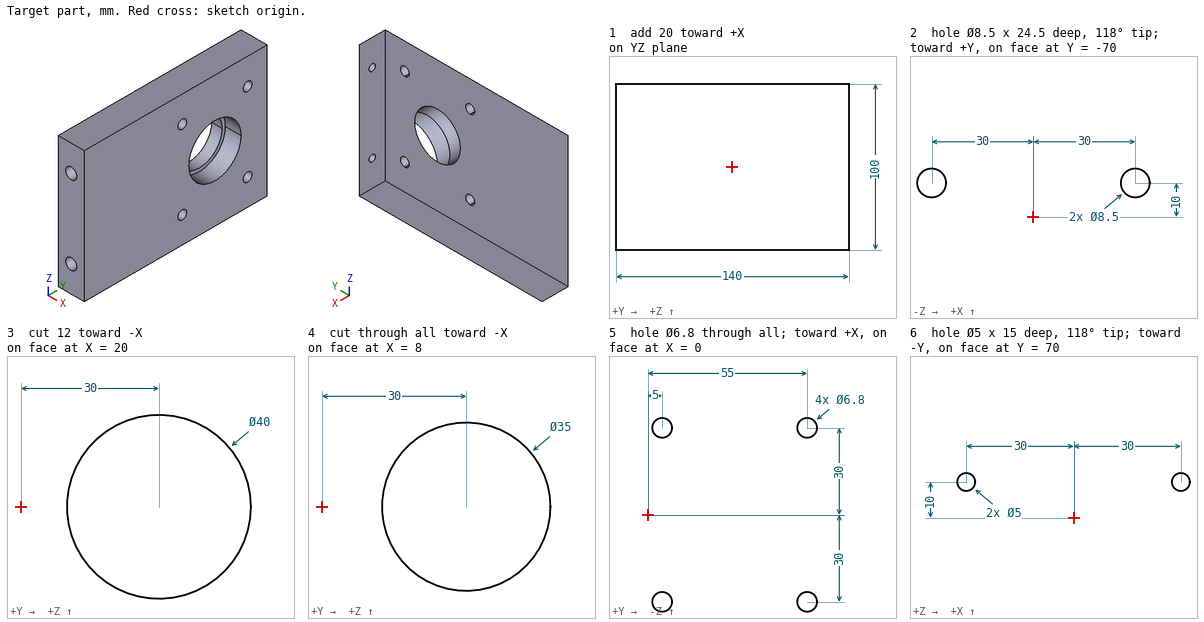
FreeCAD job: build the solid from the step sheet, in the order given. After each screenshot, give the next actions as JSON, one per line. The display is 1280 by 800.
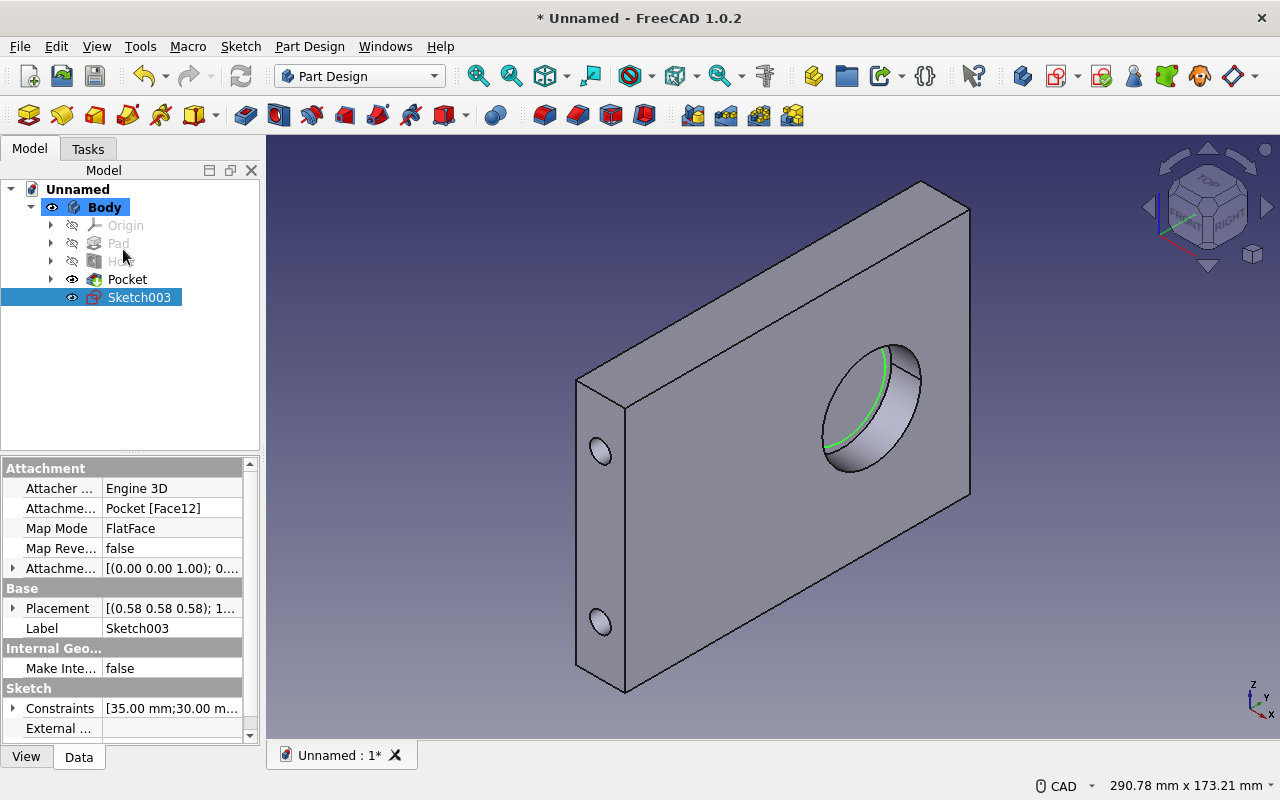
{"action": "left_click", "coordinate": [246, 116]}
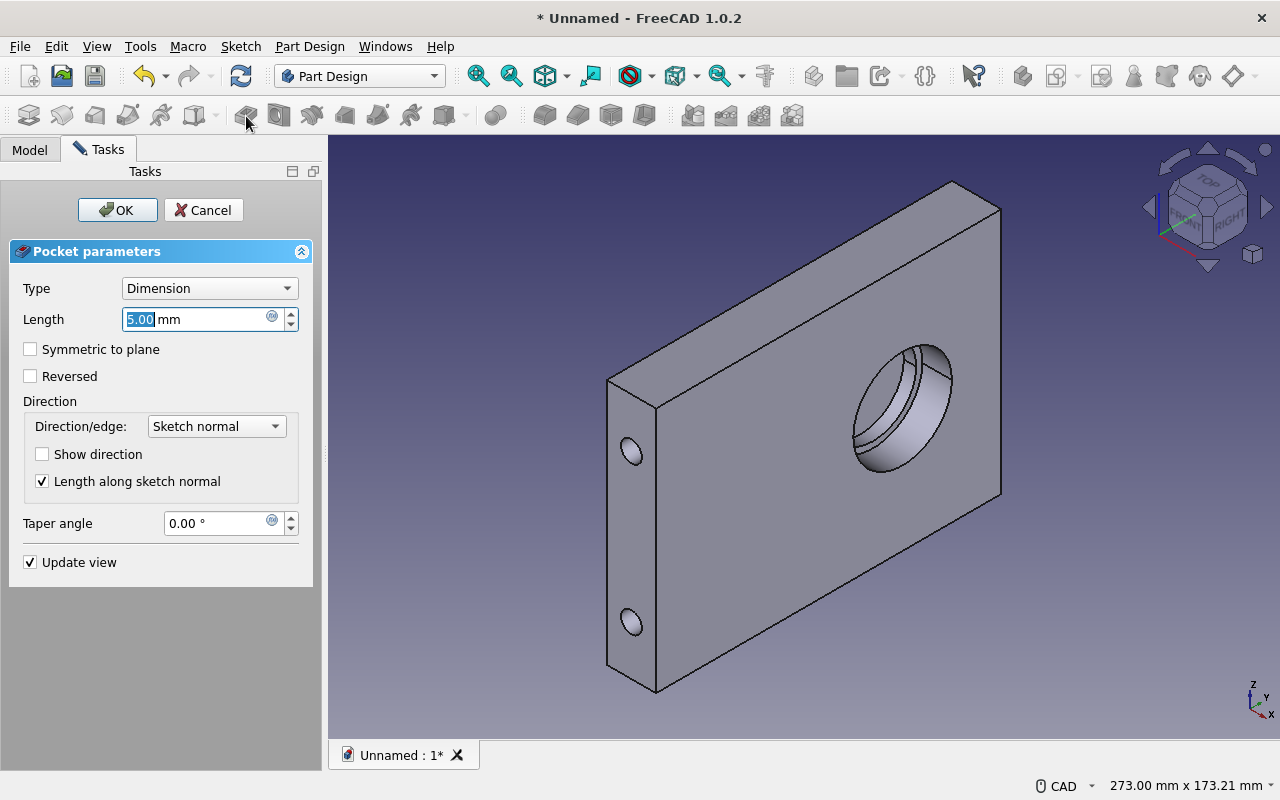
{"action": "left_click", "coordinate": [210, 288]}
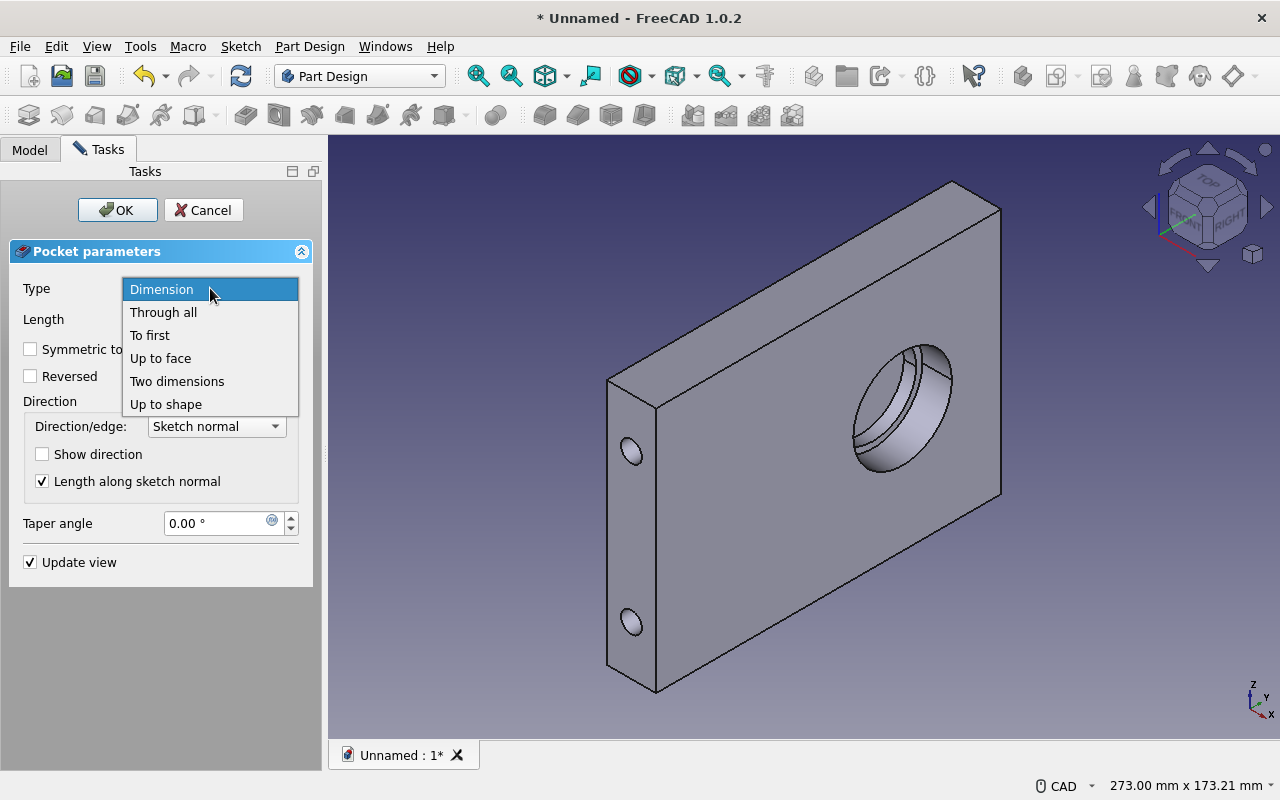
{"action": "left_click", "coordinate": [208, 312]}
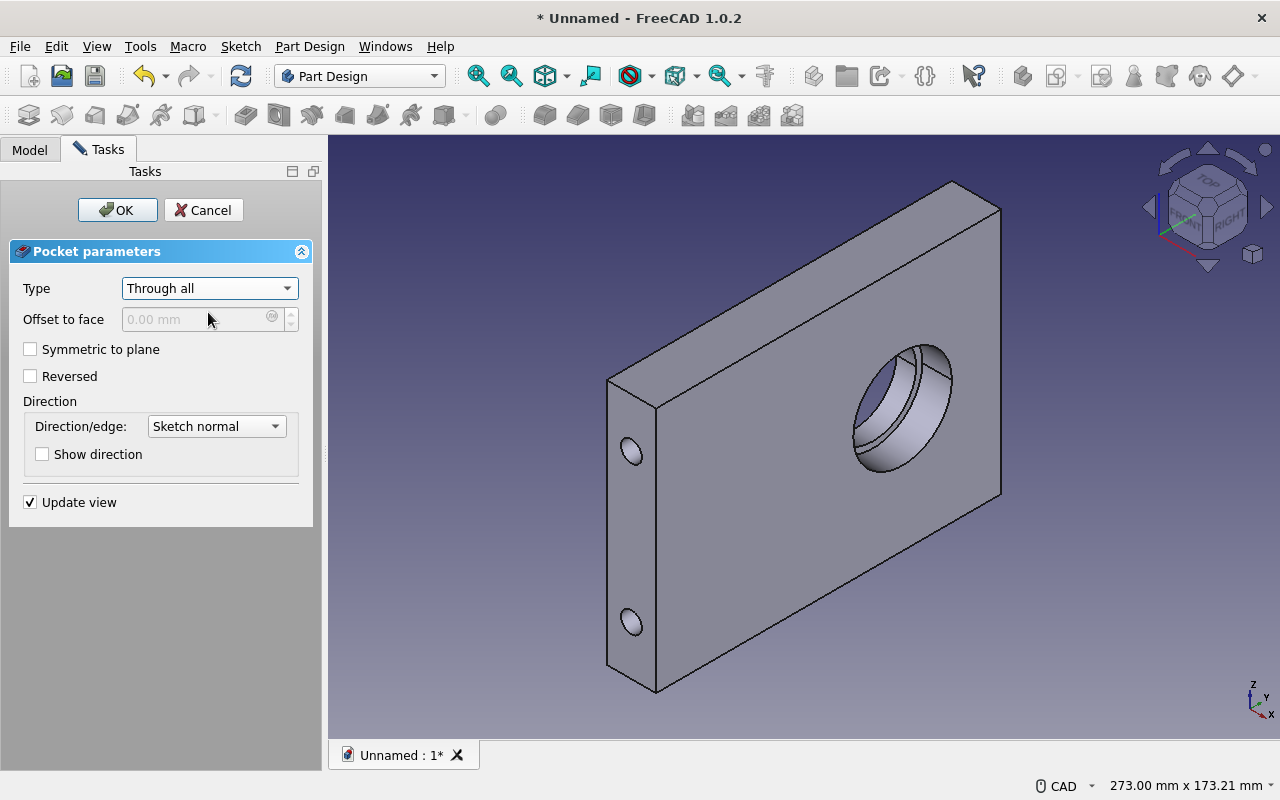
{"action": "left_click", "coordinate": [118, 210]}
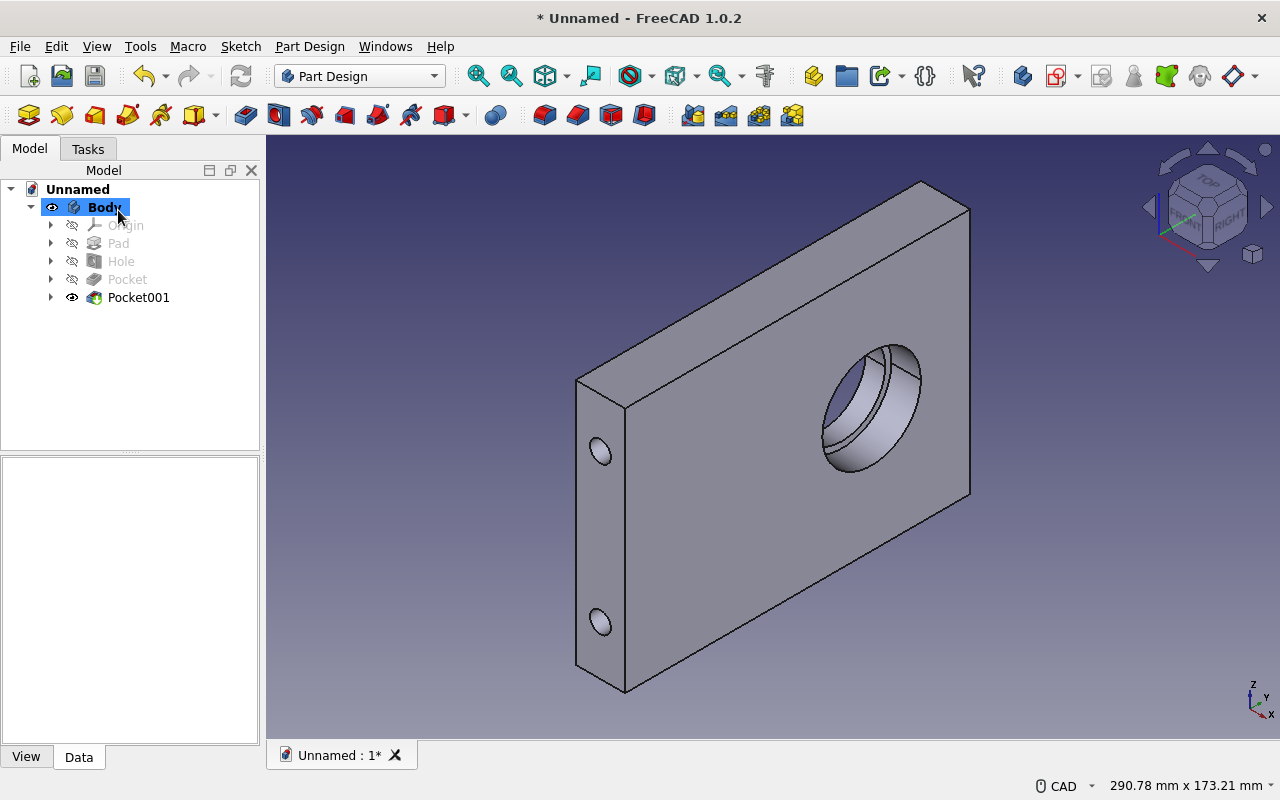
{"action": "key", "text": "6"}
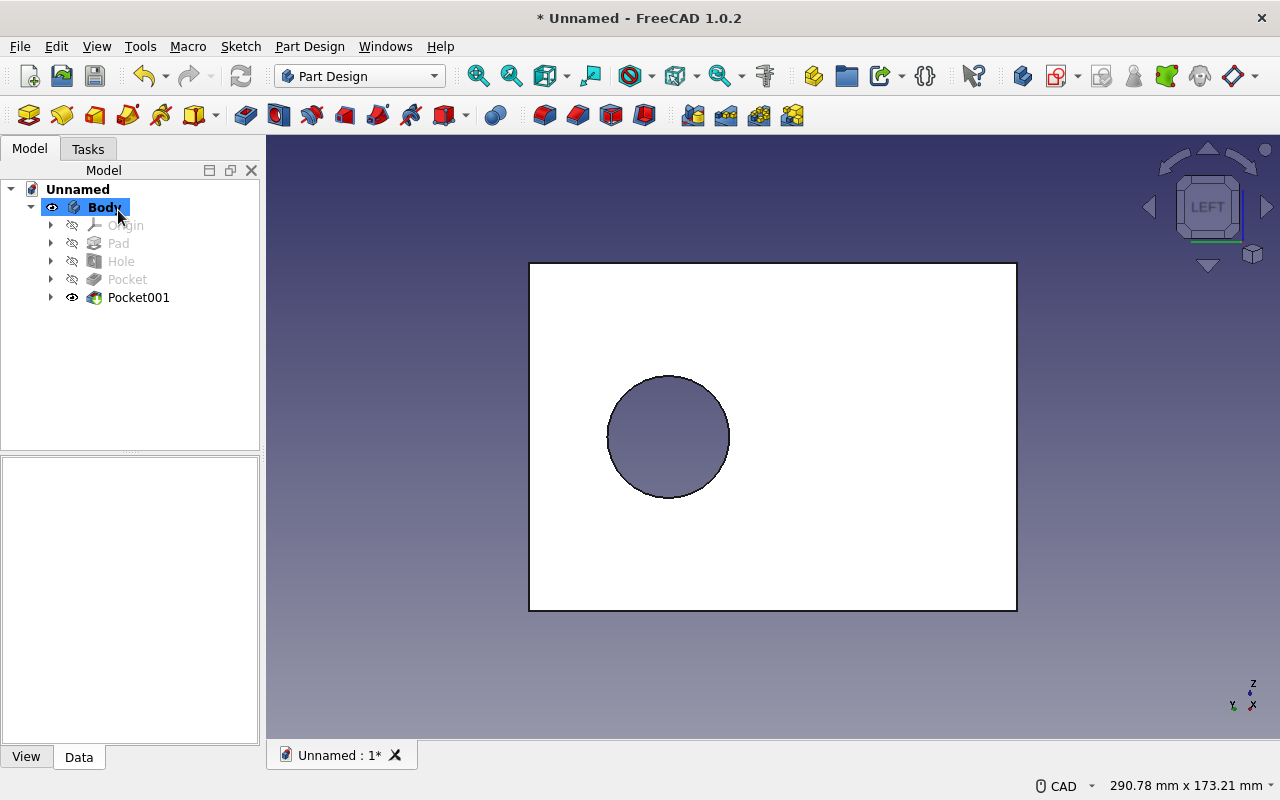
{"action": "left_click", "coordinate": [843, 386]}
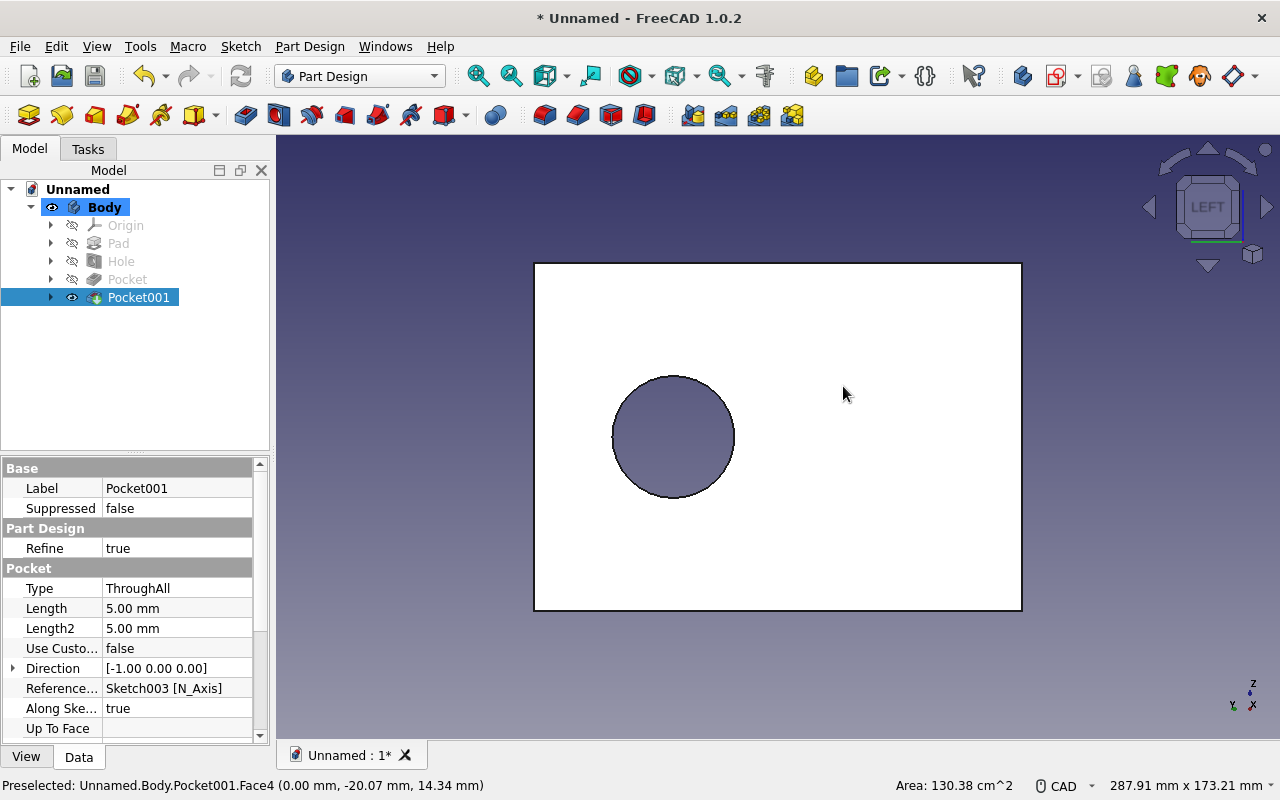
{"action": "left_click", "coordinate": [1056, 76]}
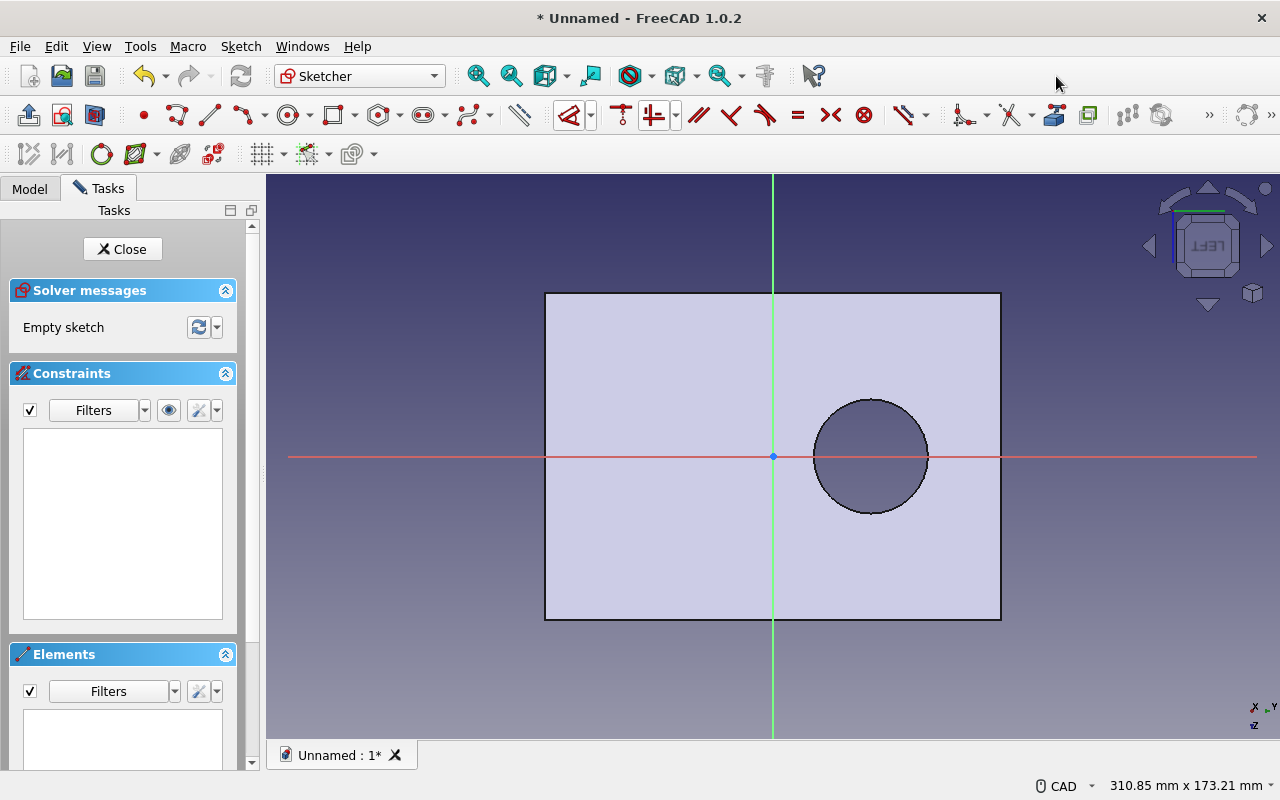
{"action": "scroll", "coordinate": [1115, 457], "scroll_direction": "up", "scroll_amount": 2}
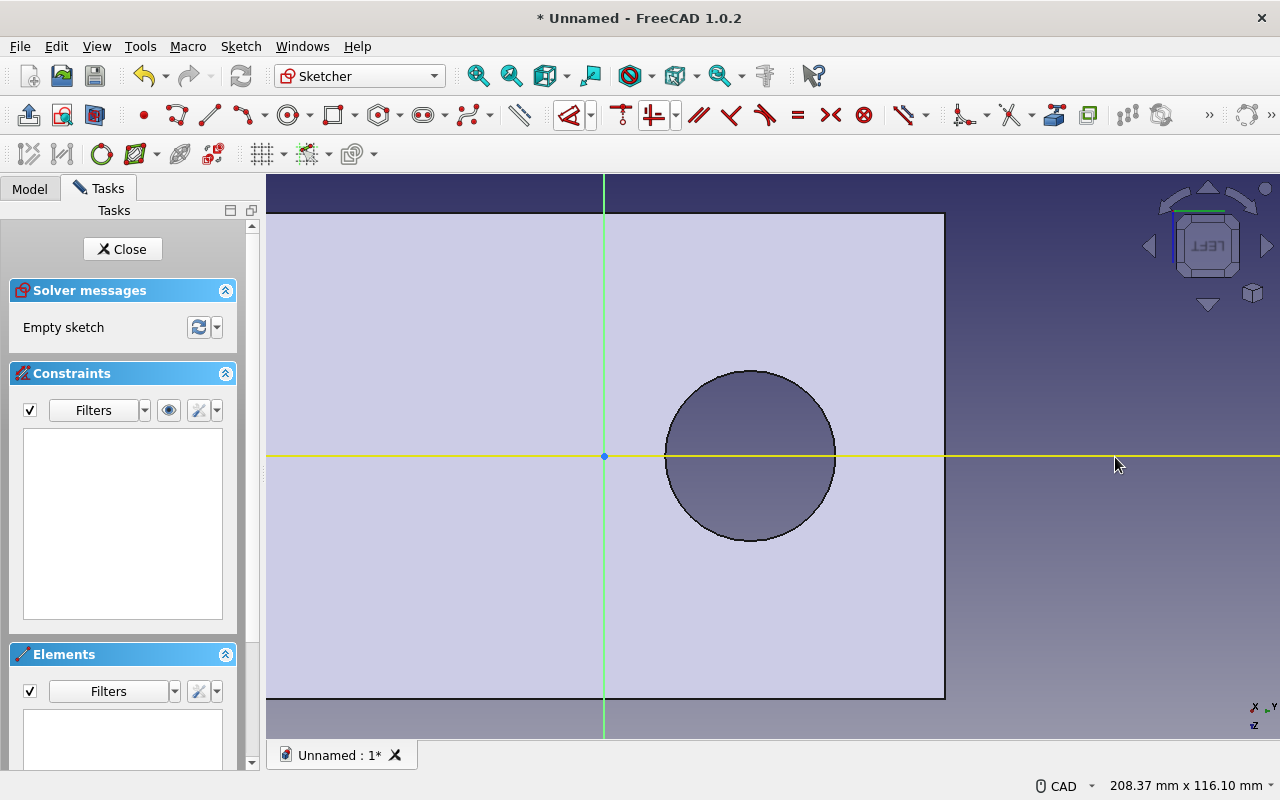
{"action": "key", "text": "g c"}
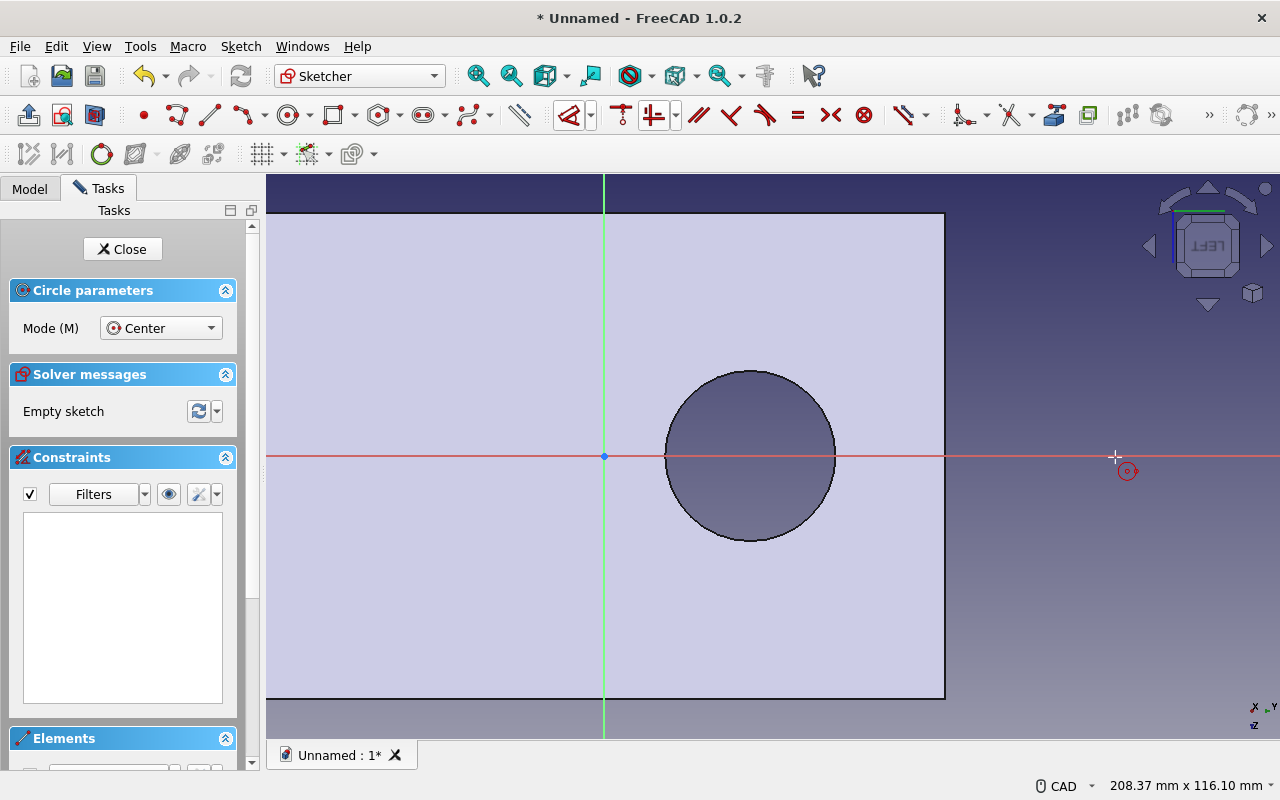
{"action": "scroll", "coordinate": [872, 310], "scroll_direction": "up", "scroll_amount": 2}